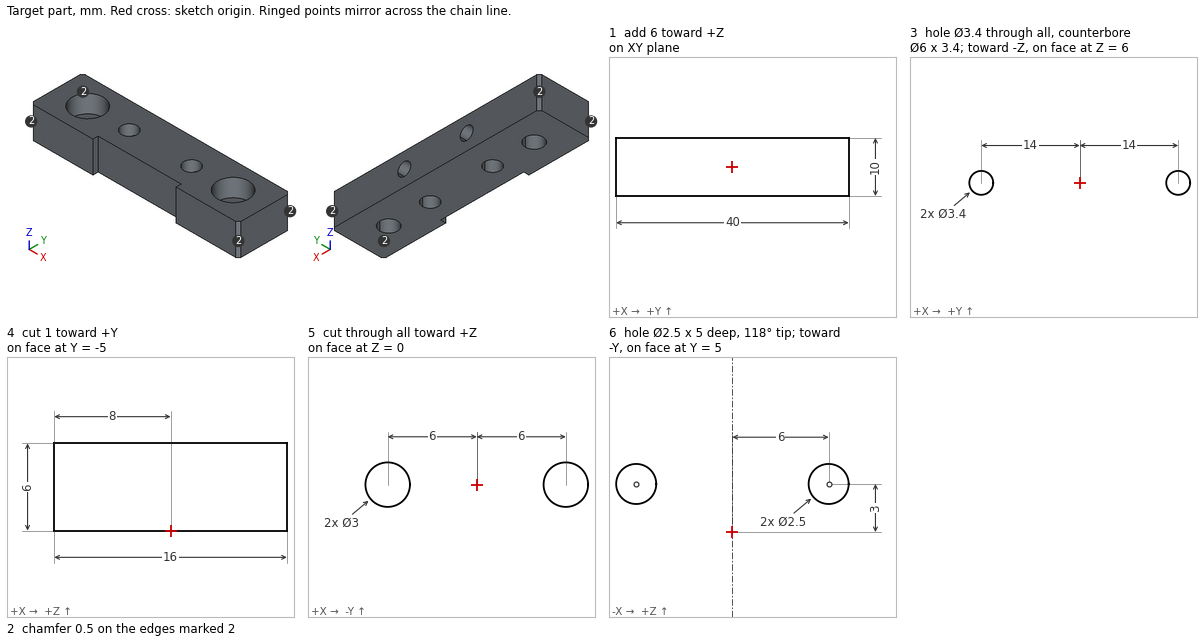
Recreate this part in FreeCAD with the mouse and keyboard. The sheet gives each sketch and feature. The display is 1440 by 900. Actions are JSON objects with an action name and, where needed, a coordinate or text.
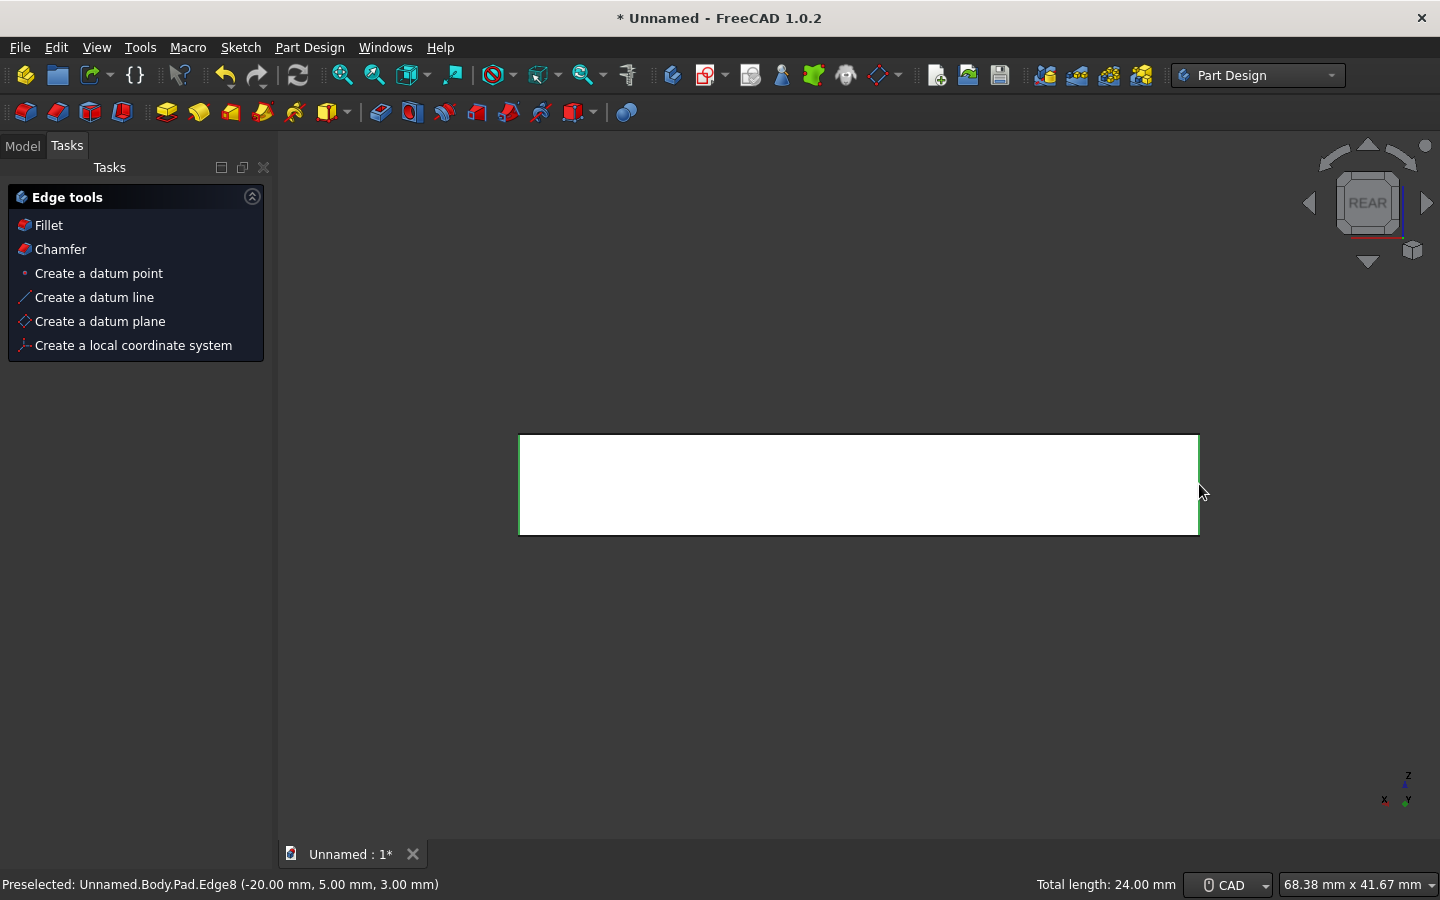
{"action": "left_click", "coordinate": [58, 112]}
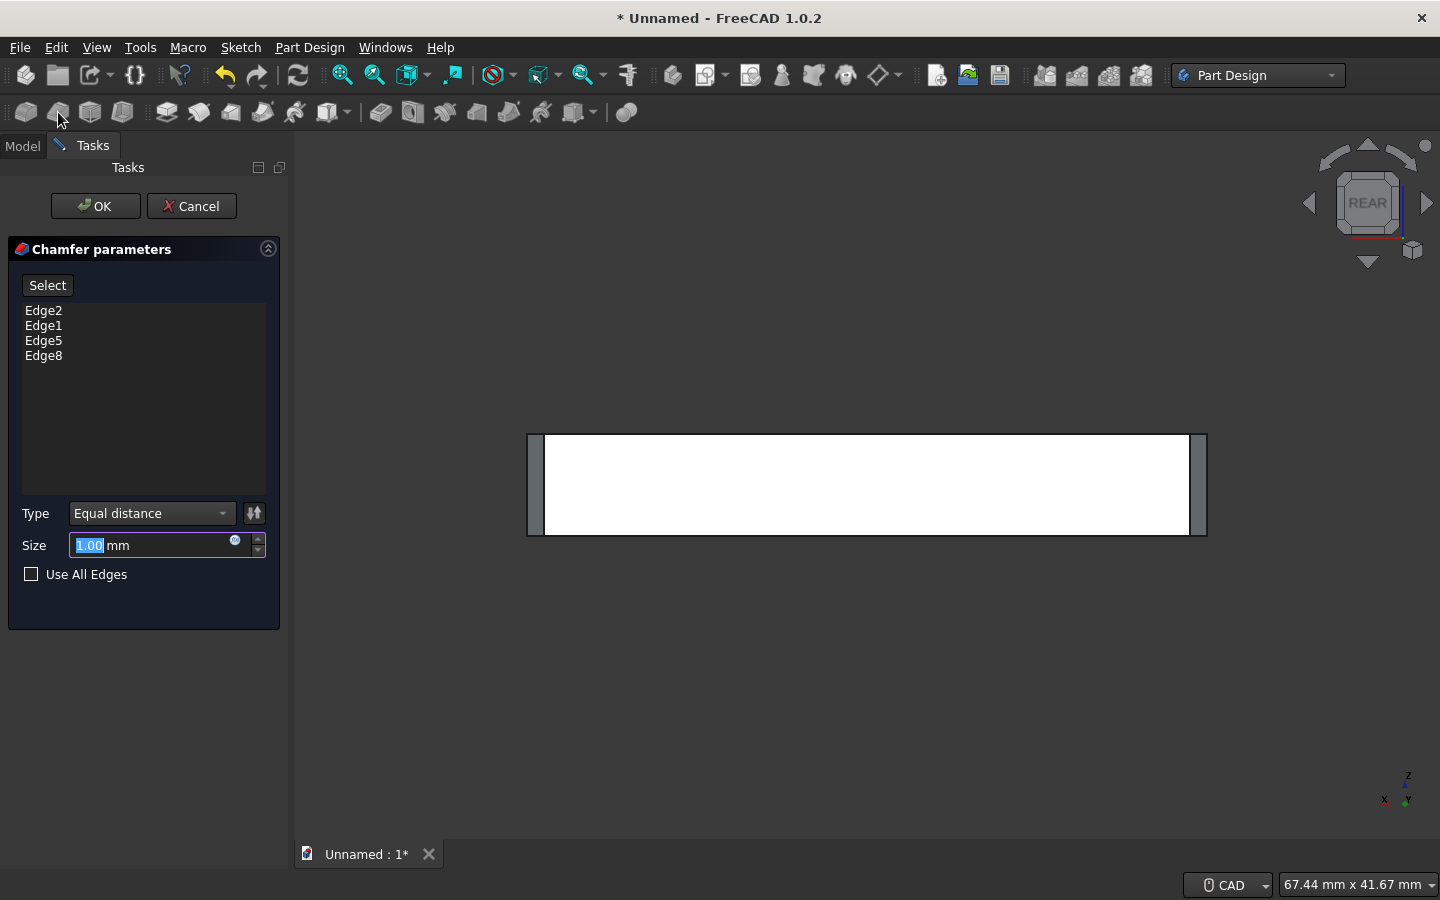
{"action": "type", "text": "0.5"}
{"action": "key", "text": "Tab"}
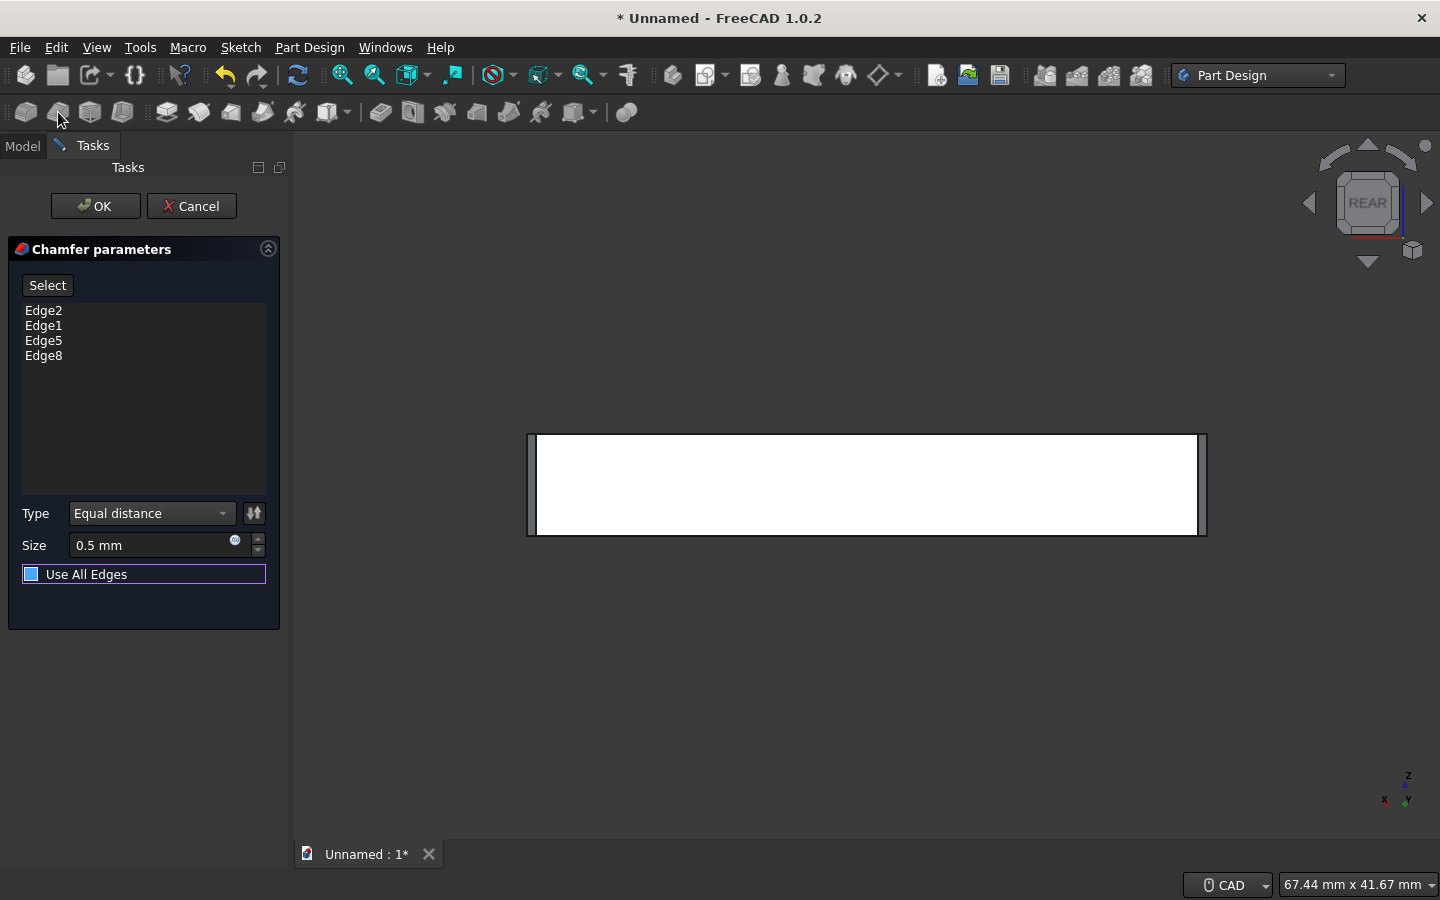
{"action": "left_click", "coordinate": [96, 206]}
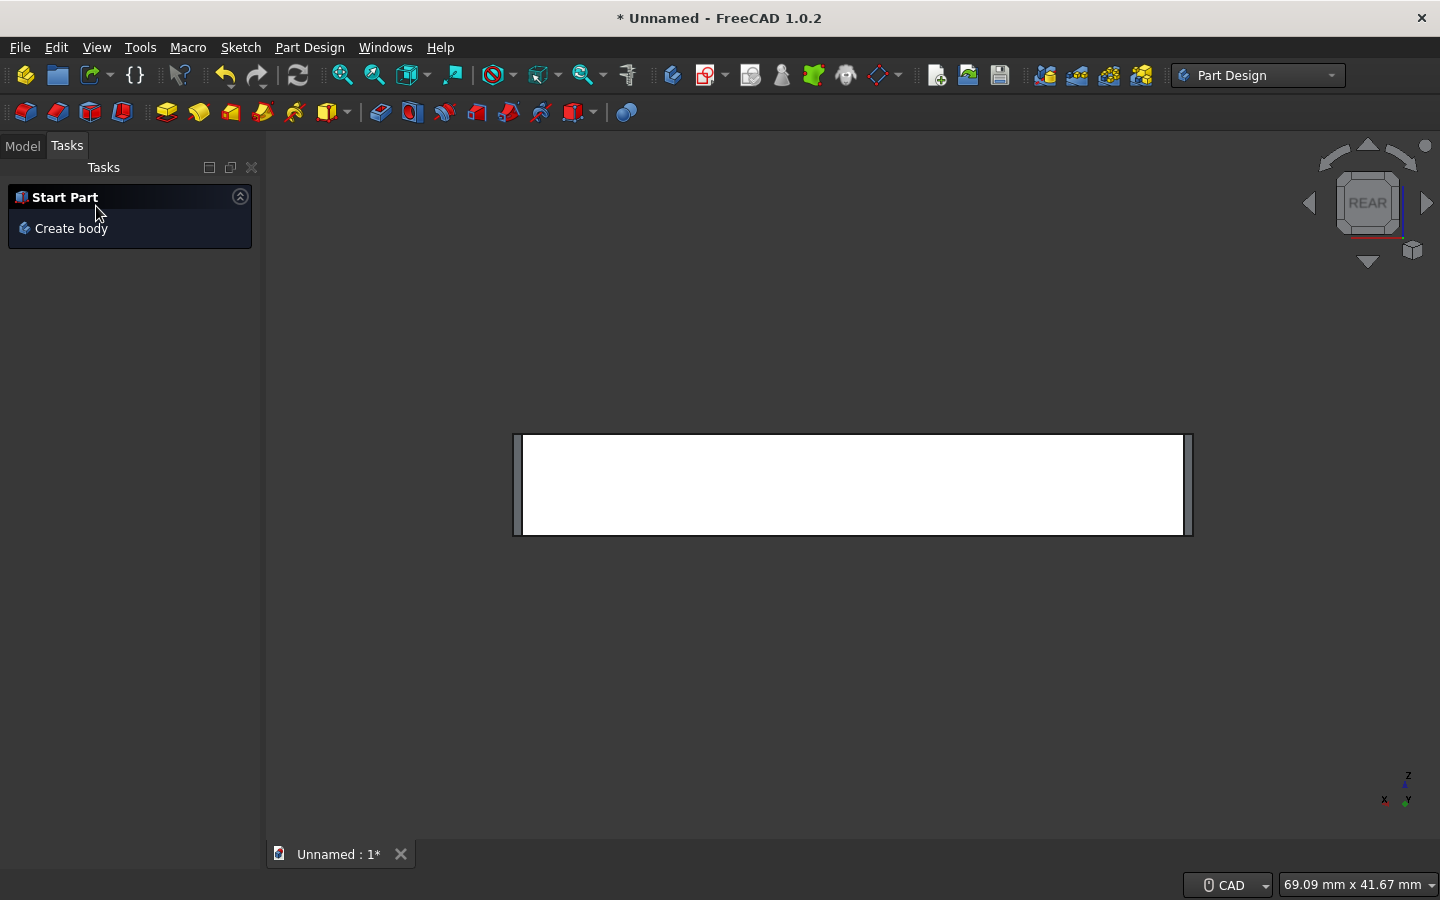
{"action": "key", "text": "0"}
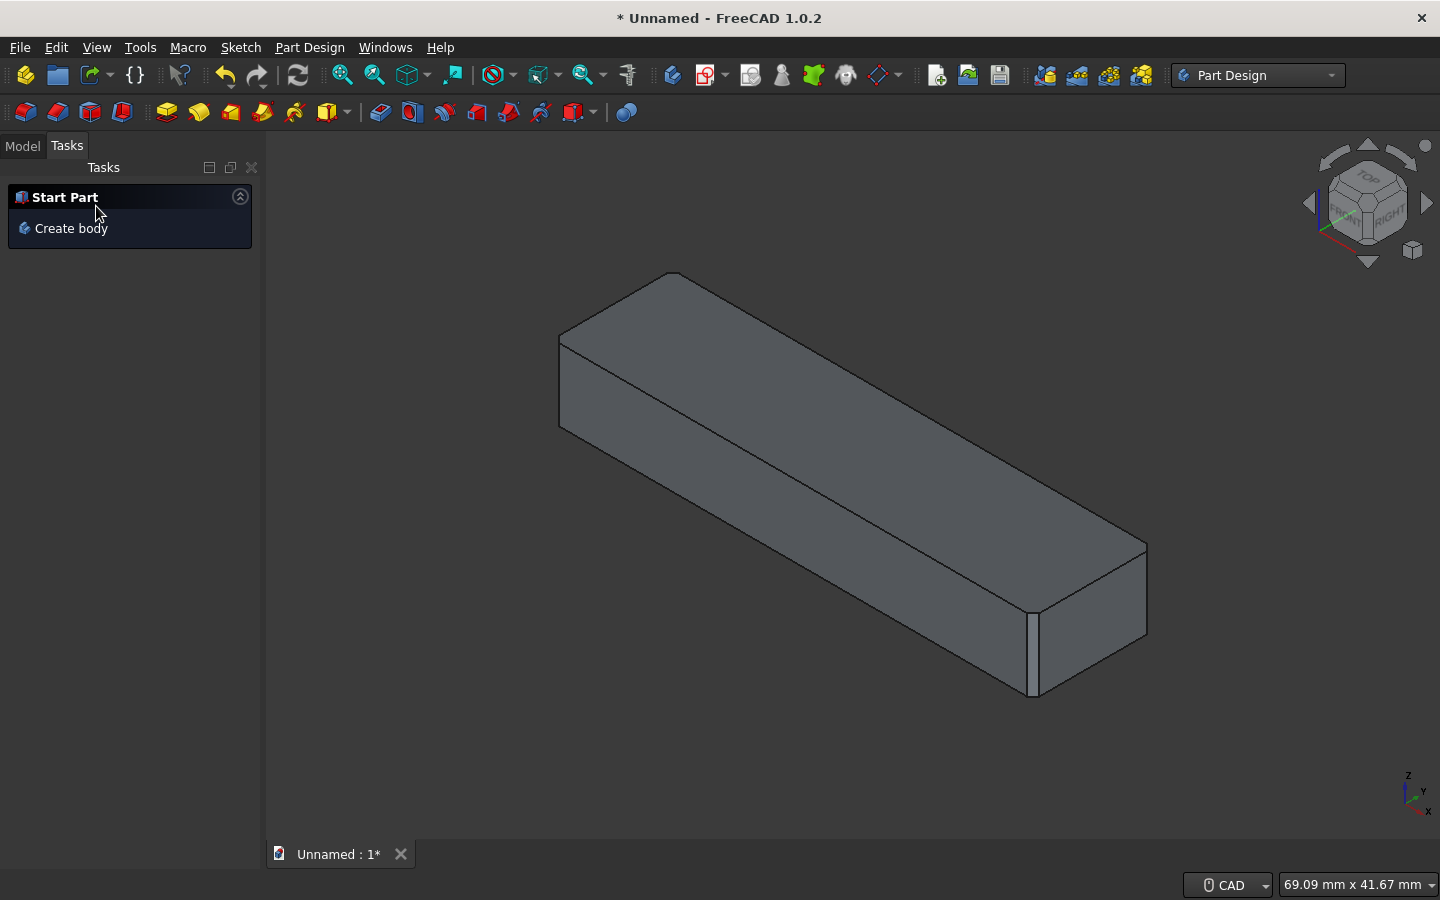
{"action": "left_click", "coordinate": [990, 522]}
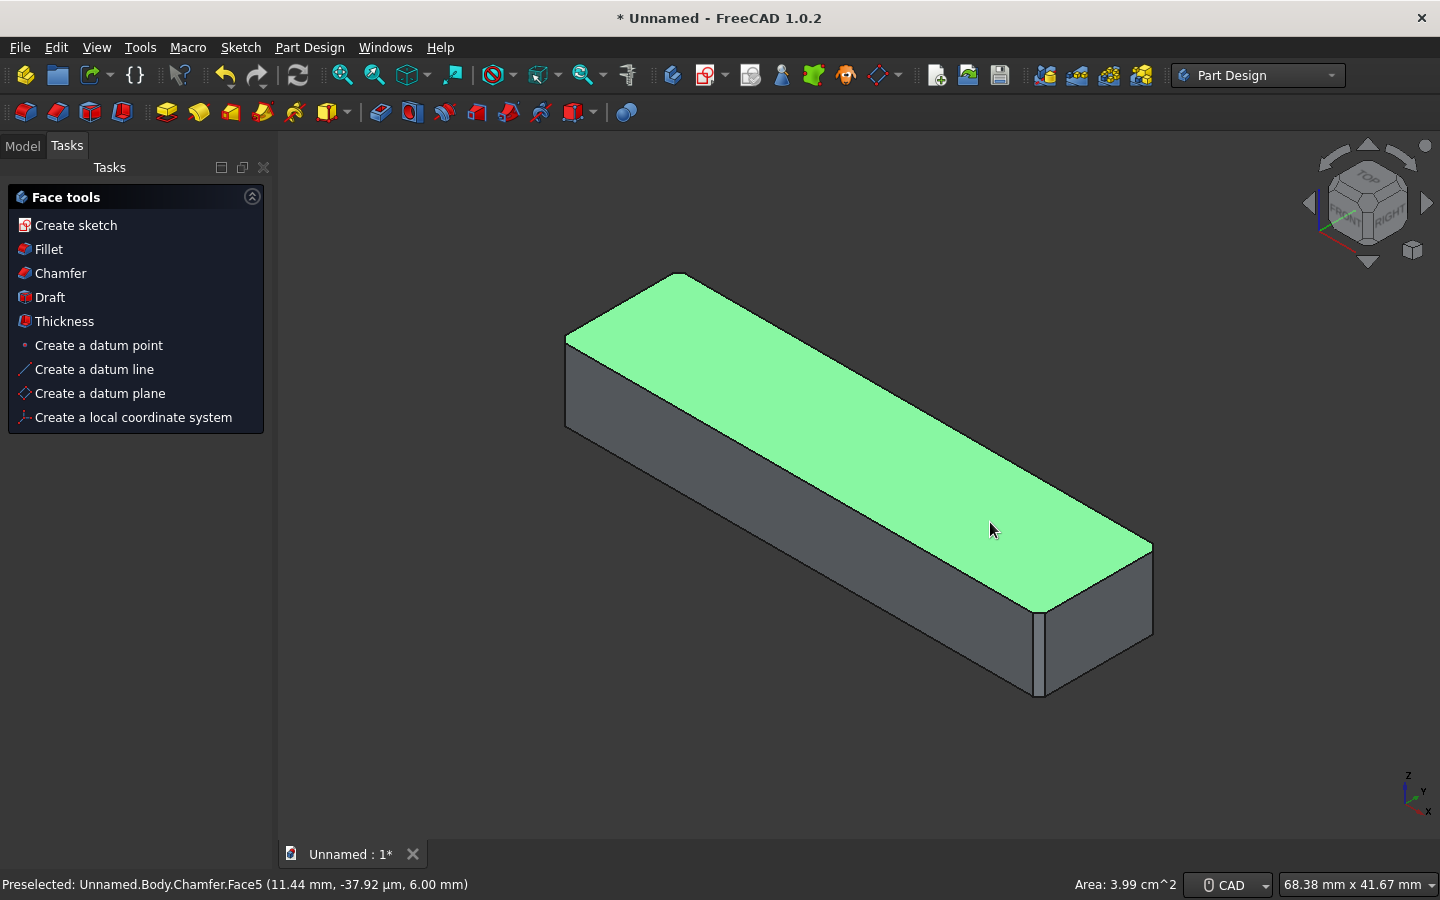
{"action": "left_click", "coordinate": [706, 76]}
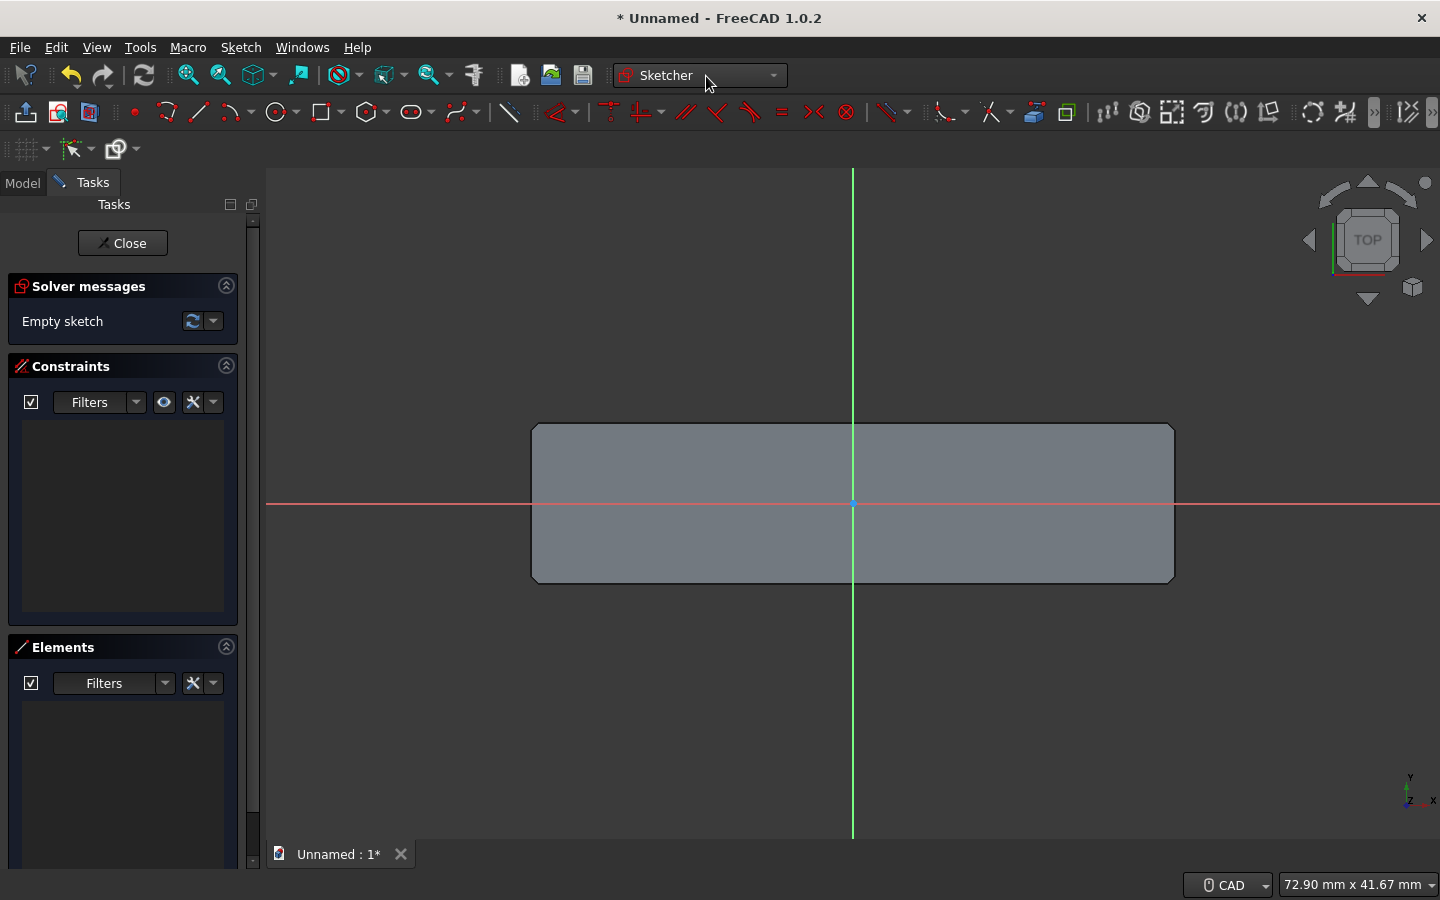
{"action": "scroll", "coordinate": [992, 504], "scroll_direction": "up", "scroll_amount": 2}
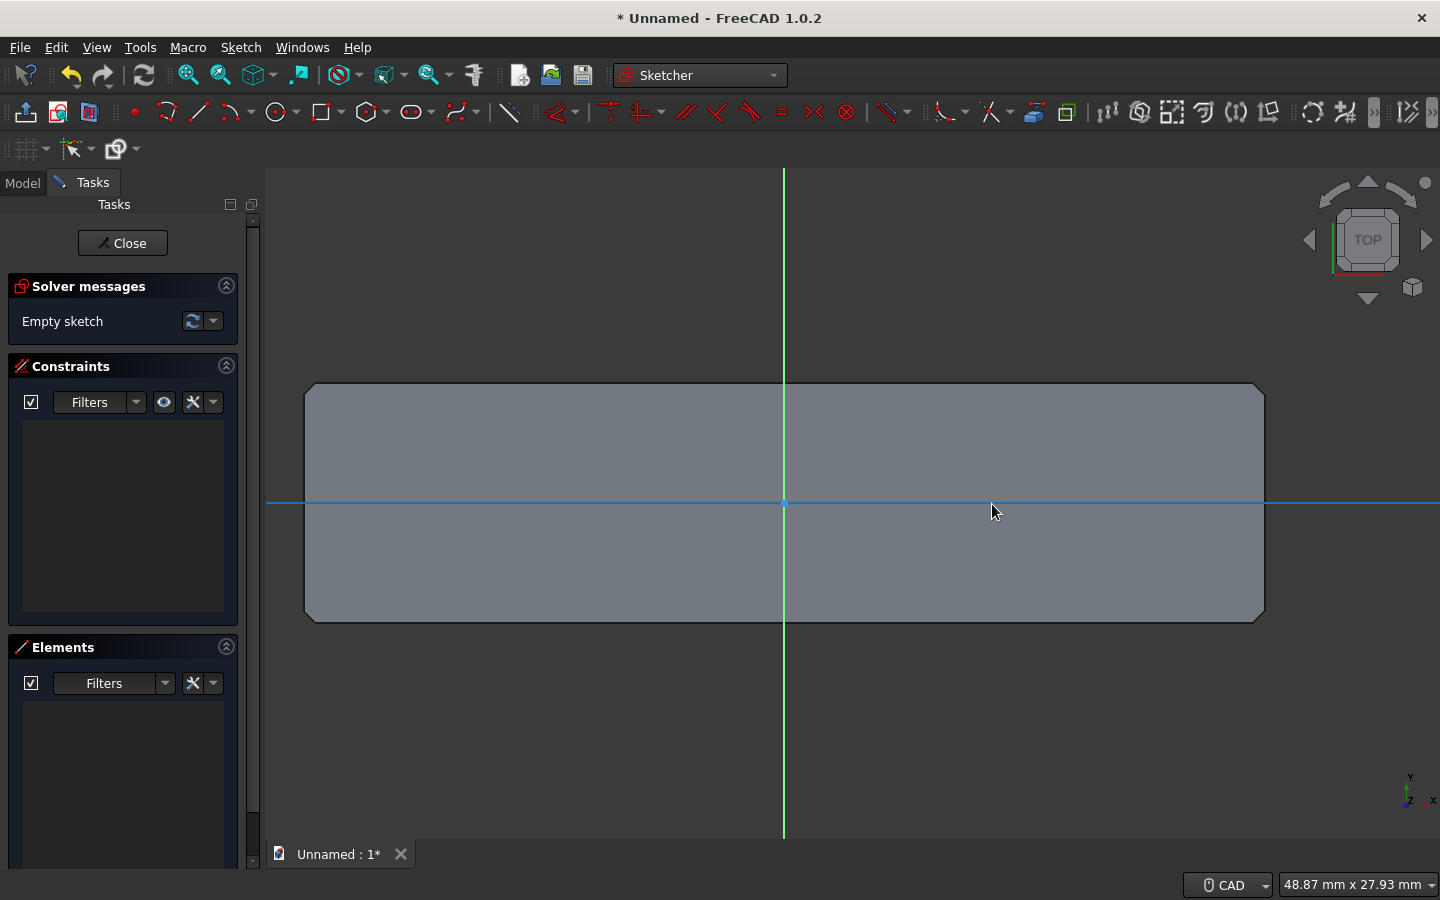
{"action": "left_click", "coordinate": [276, 112]}